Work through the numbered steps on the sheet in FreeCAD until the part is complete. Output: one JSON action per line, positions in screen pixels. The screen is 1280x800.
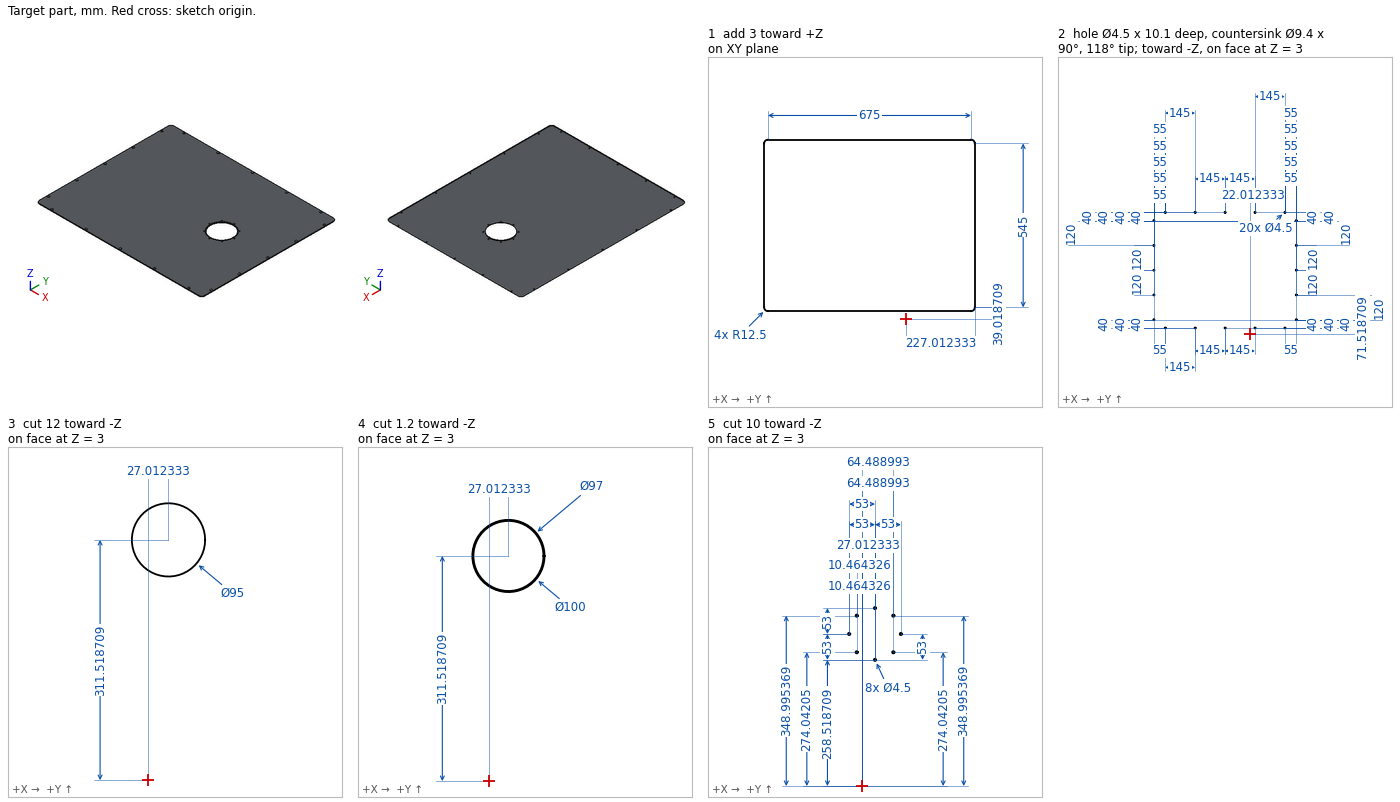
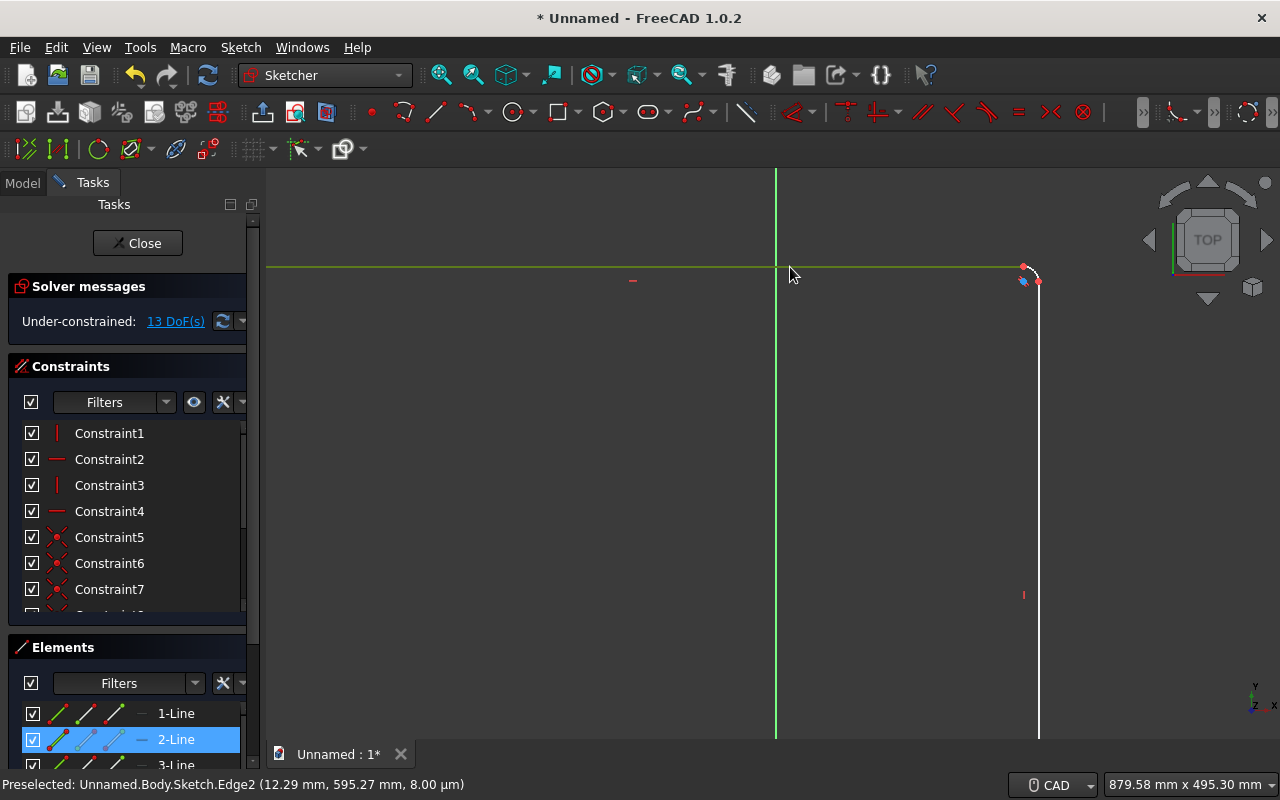
{"action": "scroll", "coordinate": [790, 264], "scroll_direction": "down", "scroll_amount": 3}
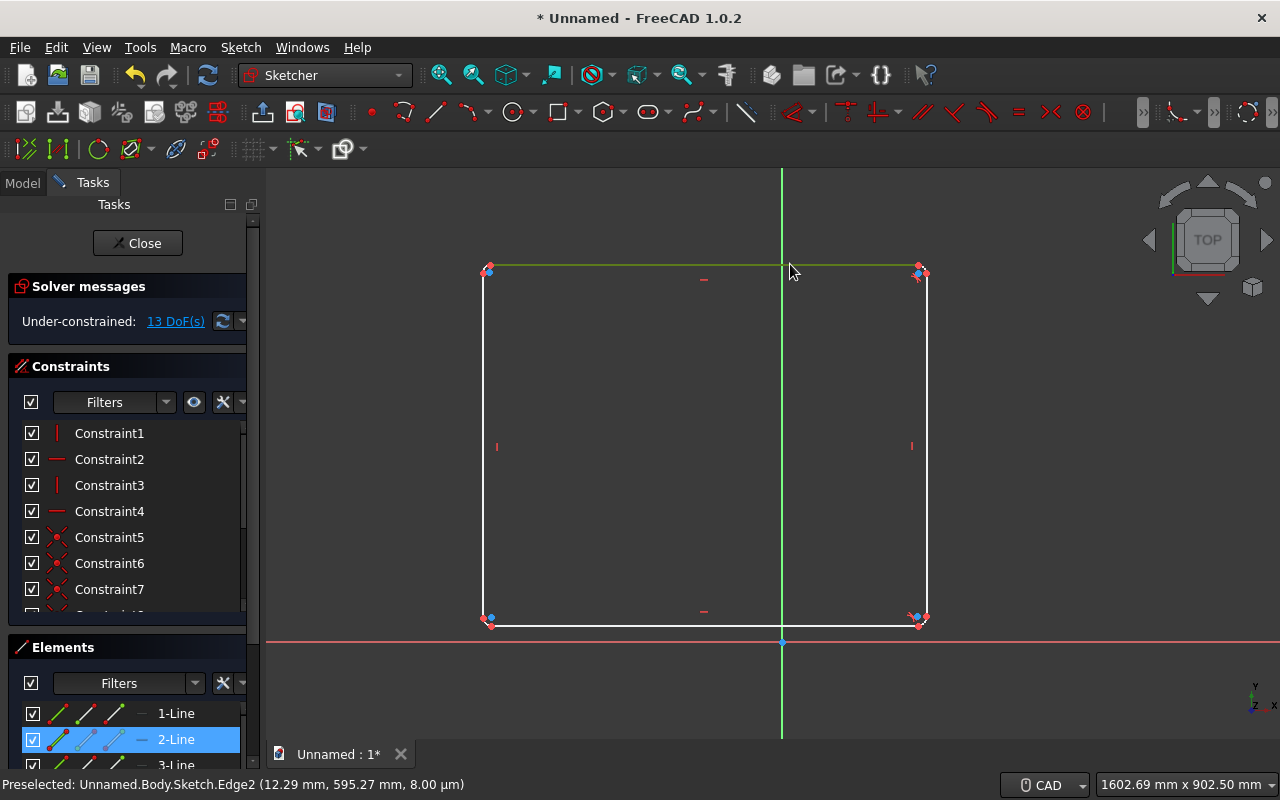
{"action": "scroll", "coordinate": [485, 268], "scroll_direction": "up", "scroll_amount": 4}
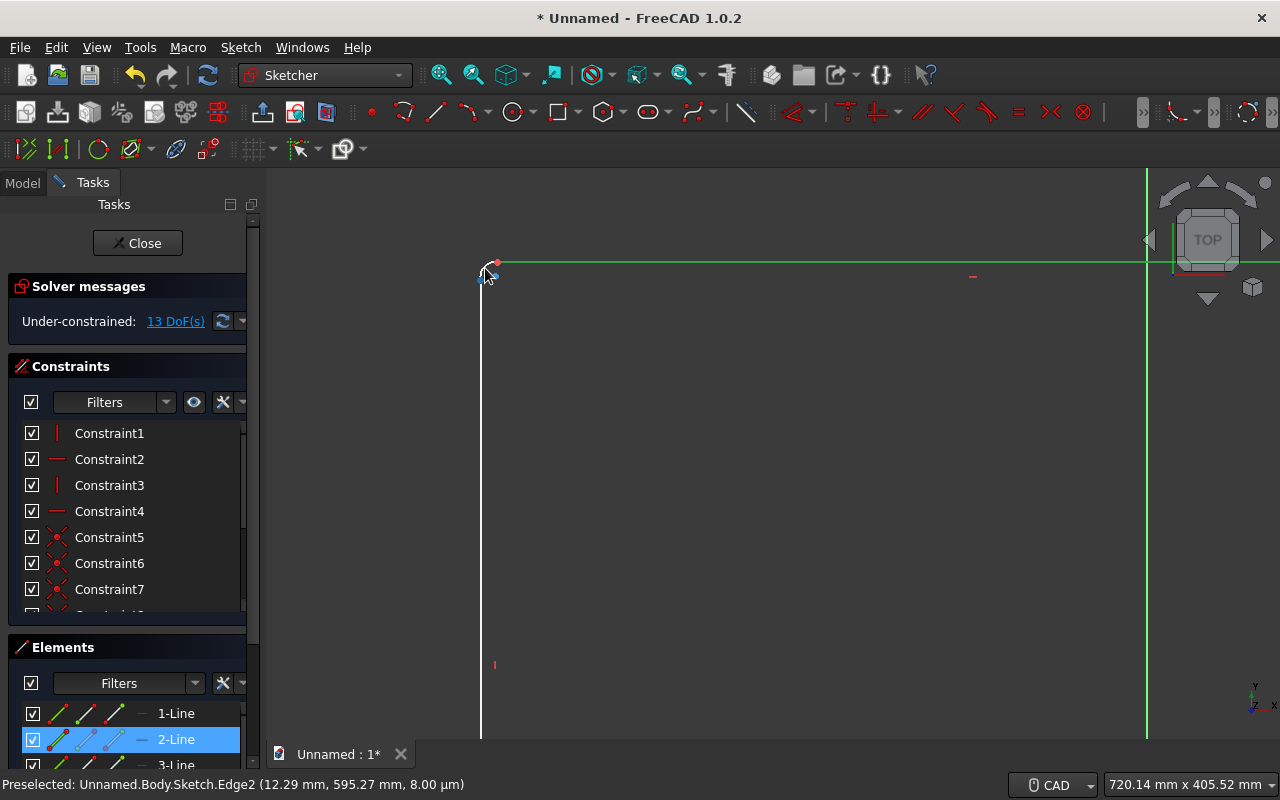
{"action": "left_click", "coordinate": [484, 267]}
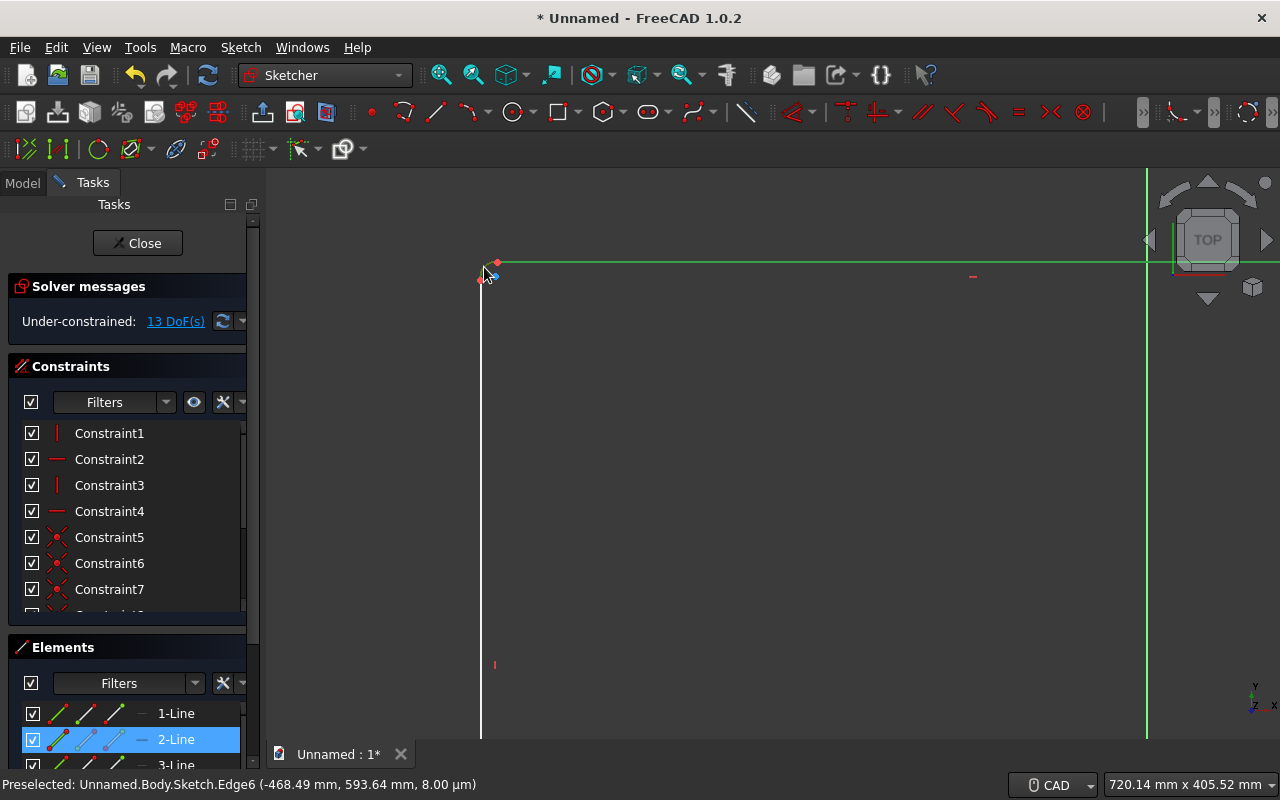
{"action": "left_click", "coordinate": [988, 112]}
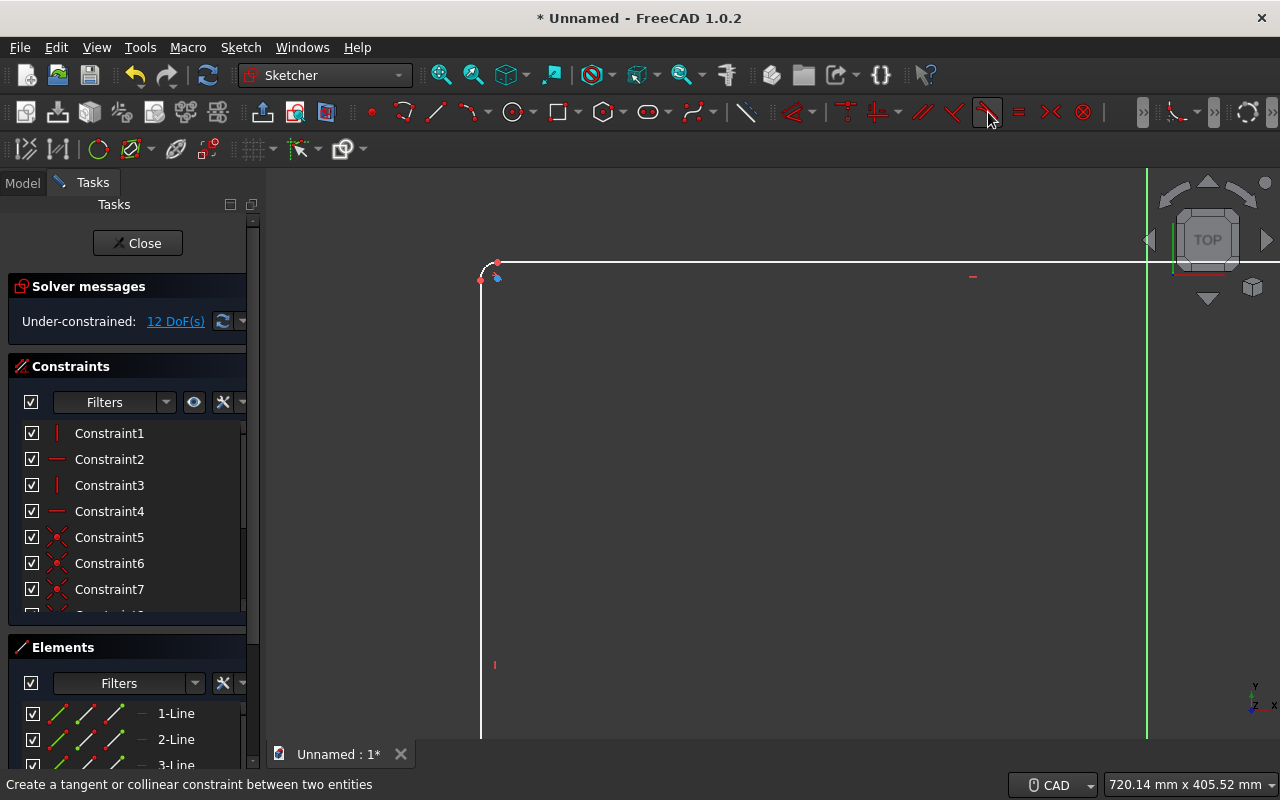
{"action": "left_click", "coordinate": [481, 511]}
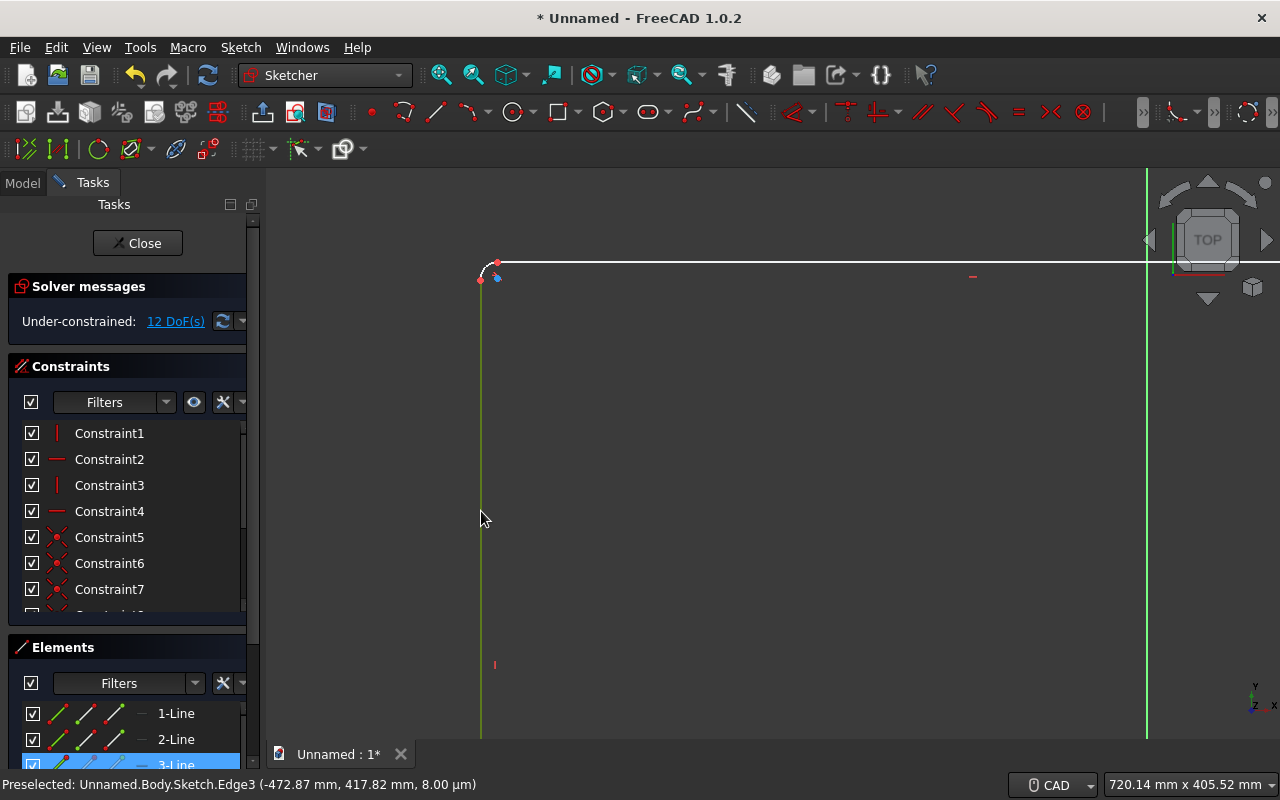
{"action": "left_click", "coordinate": [485, 268]}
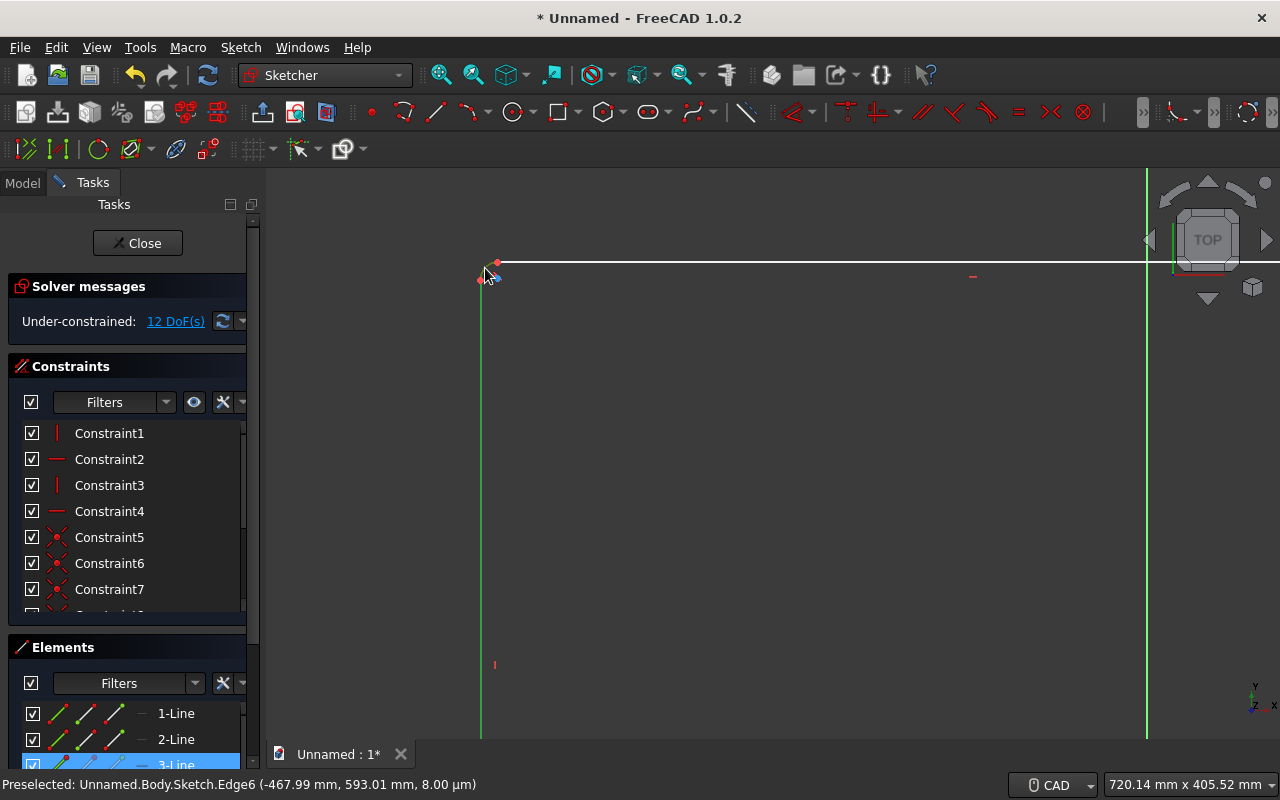
{"action": "left_click", "coordinate": [988, 112]}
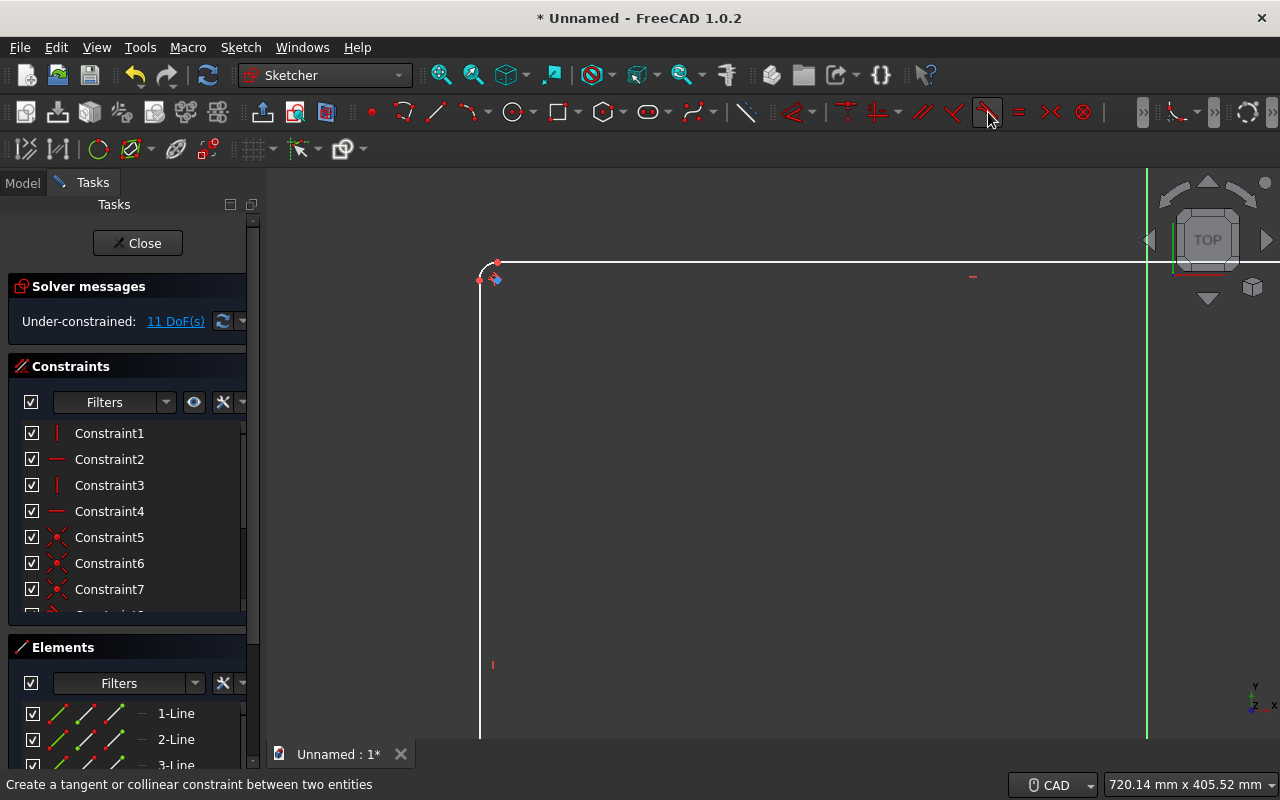
{"action": "left_click", "coordinate": [480, 511]}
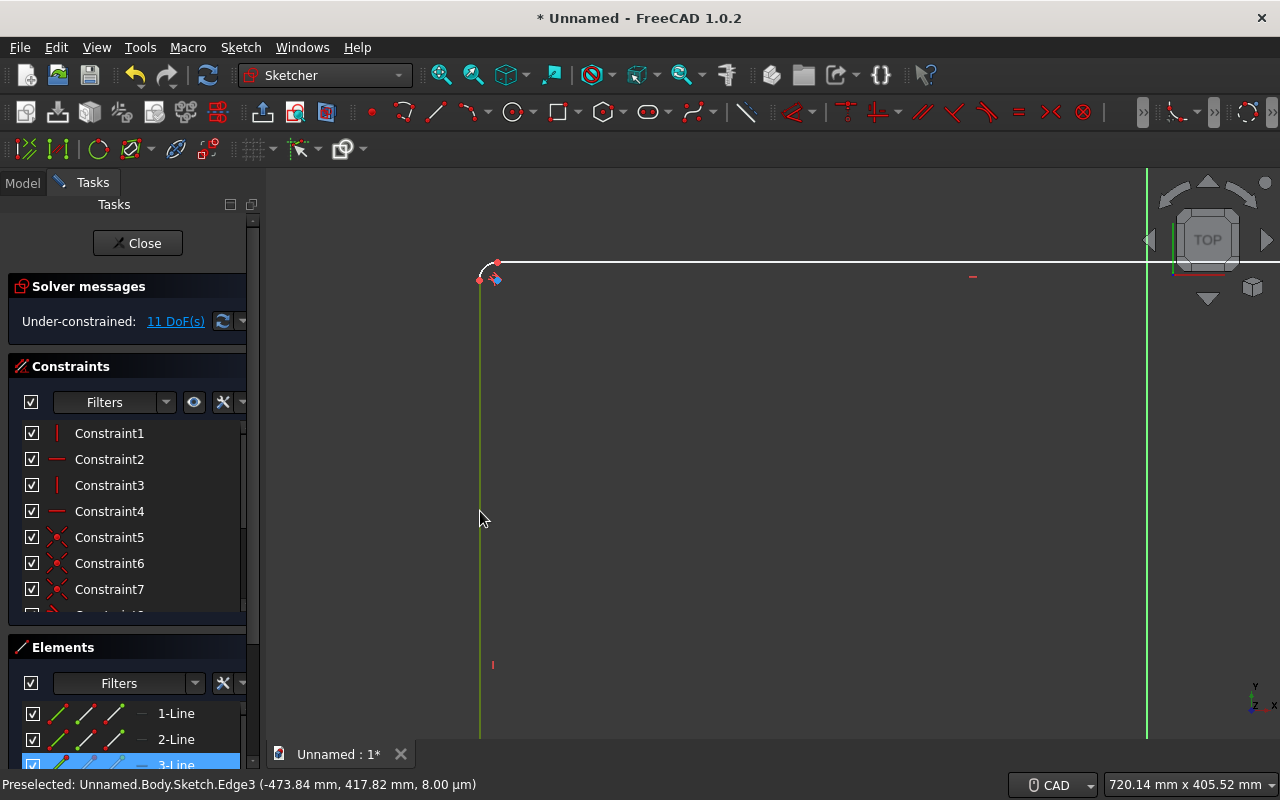
{"action": "scroll", "coordinate": [485, 268], "scroll_direction": "down", "scroll_amount": 4}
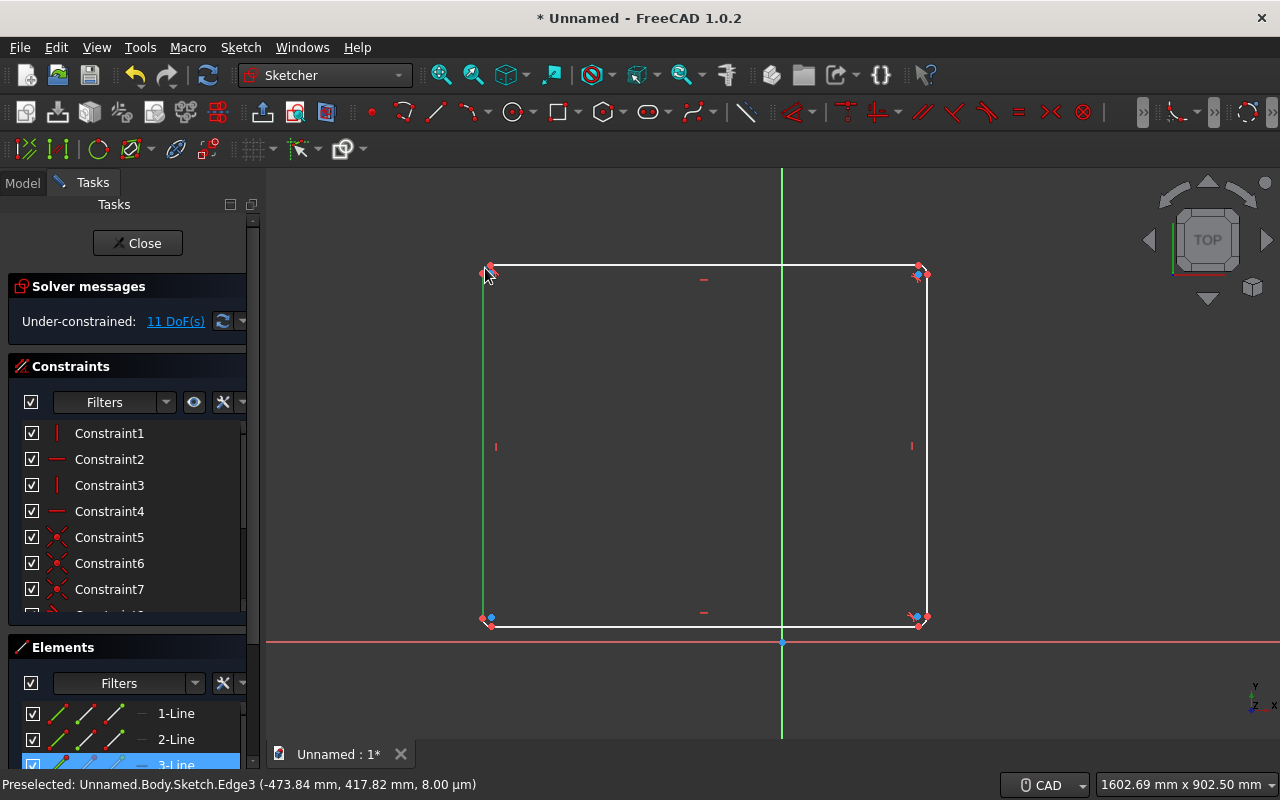
{"action": "scroll", "coordinate": [485, 624], "scroll_direction": "up", "scroll_amount": 5}